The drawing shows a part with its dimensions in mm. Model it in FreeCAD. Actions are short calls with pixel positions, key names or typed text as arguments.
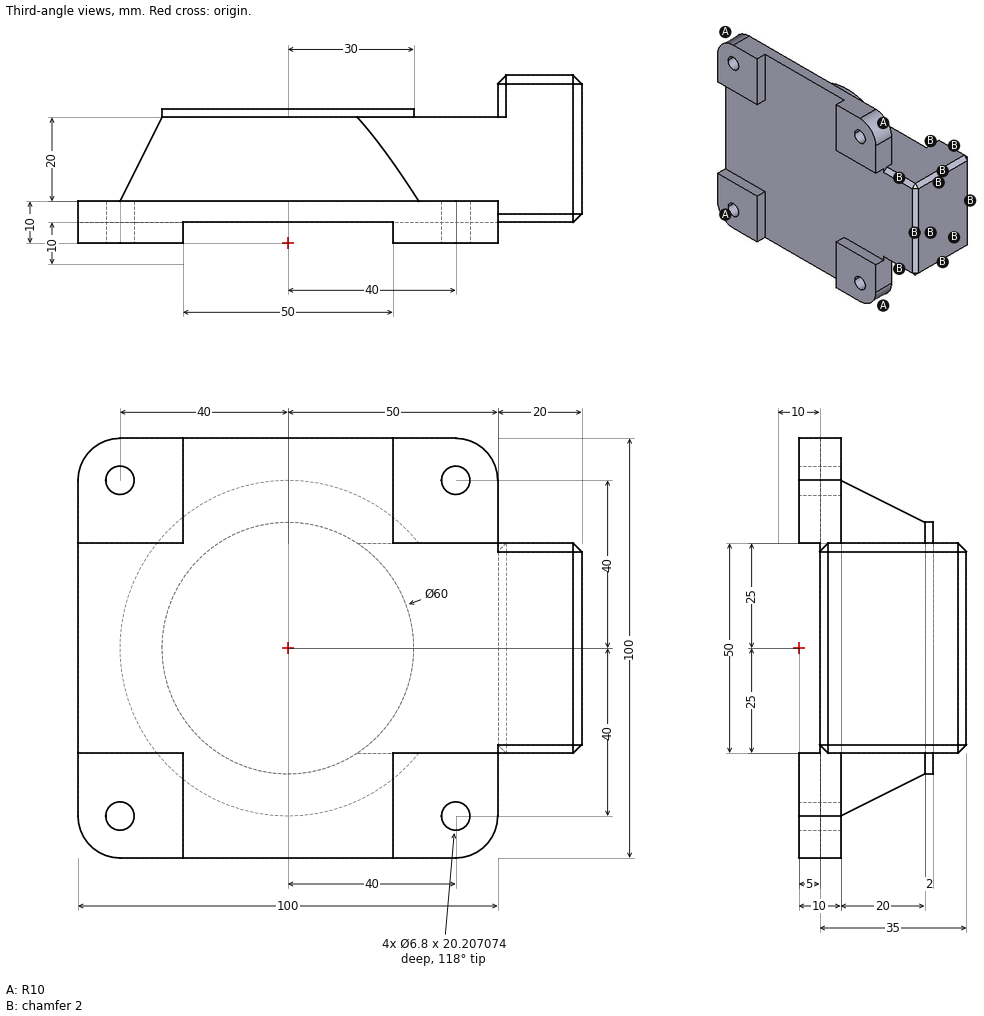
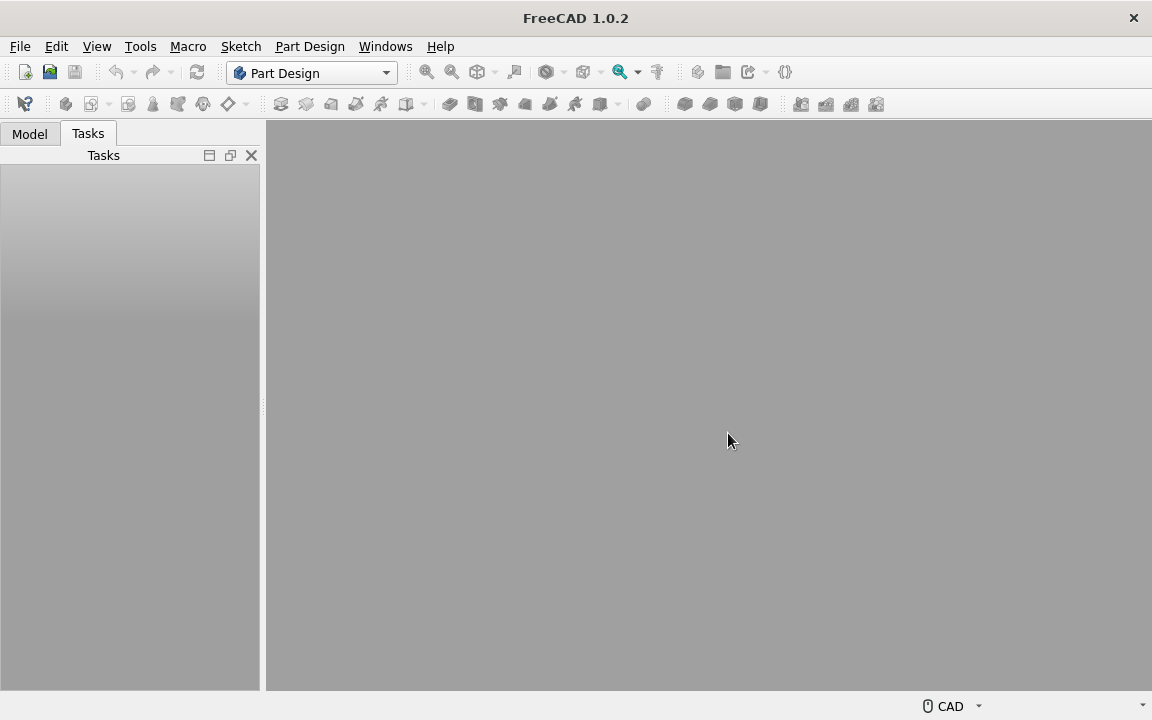
click(25, 72)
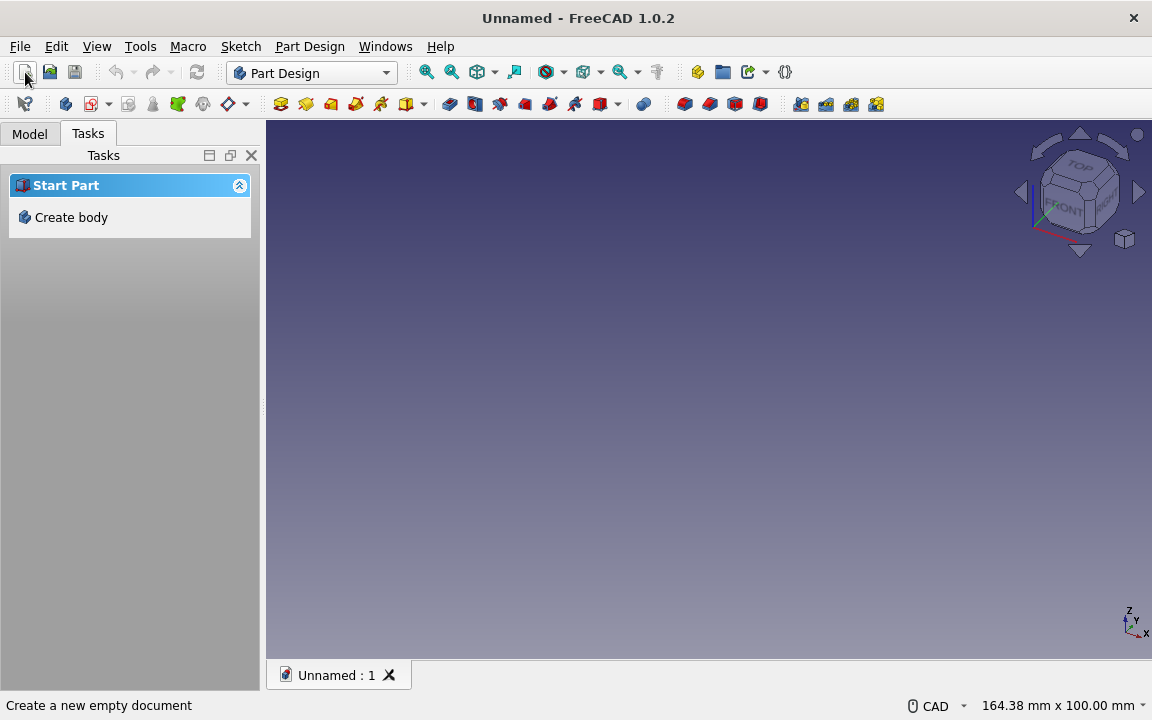
click(90, 104)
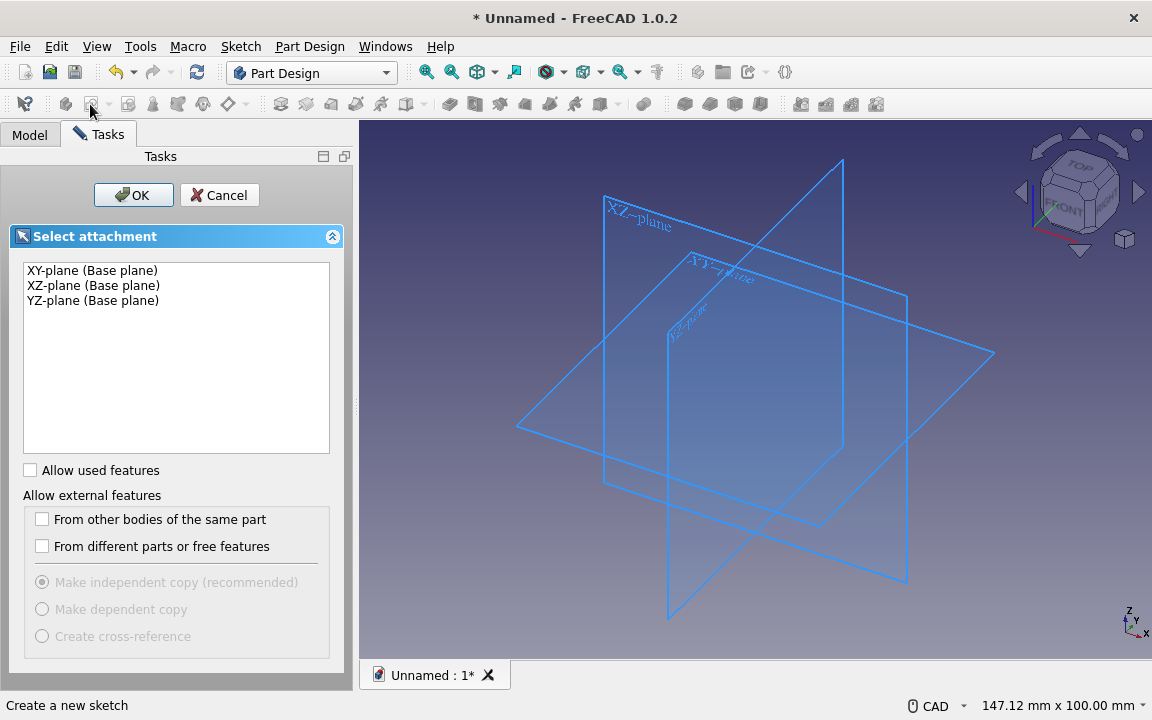
click(84, 286)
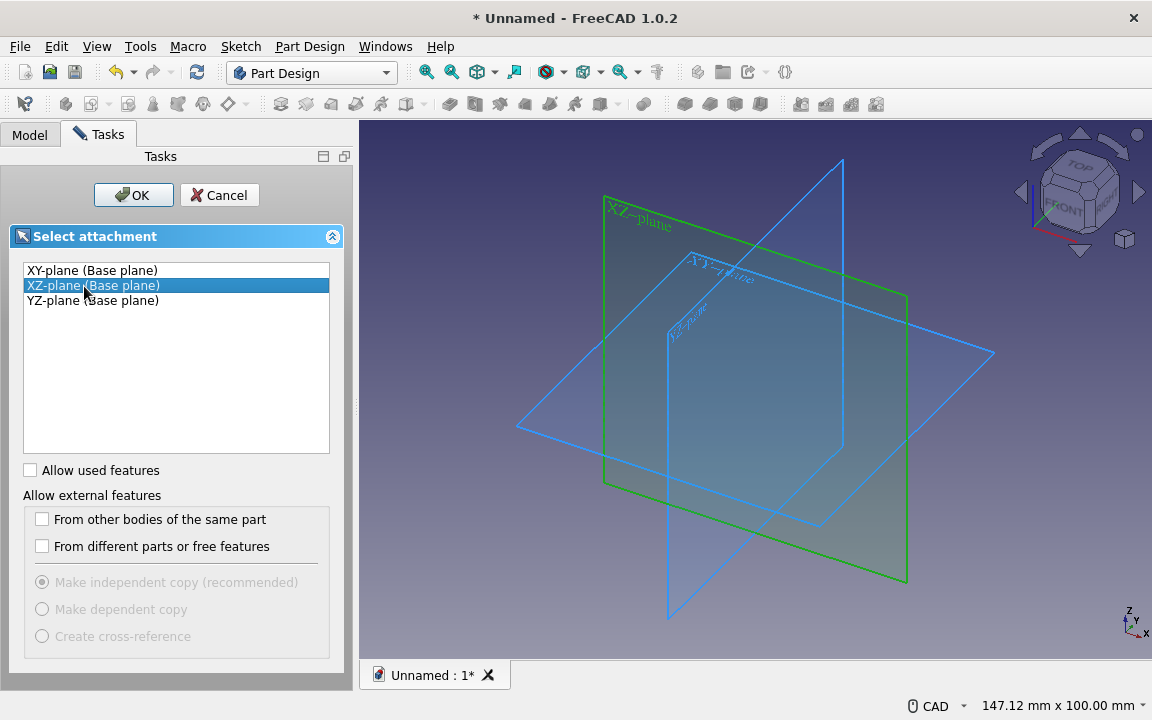
click(134, 195)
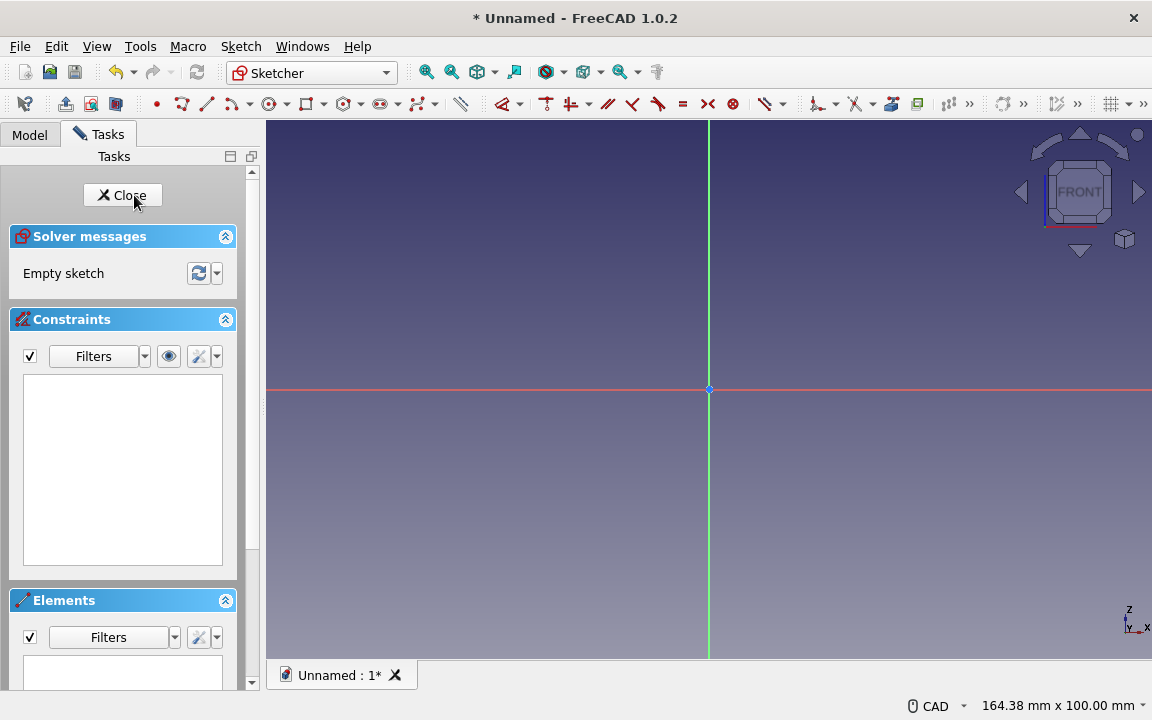
scroll(501, 390, down, 2)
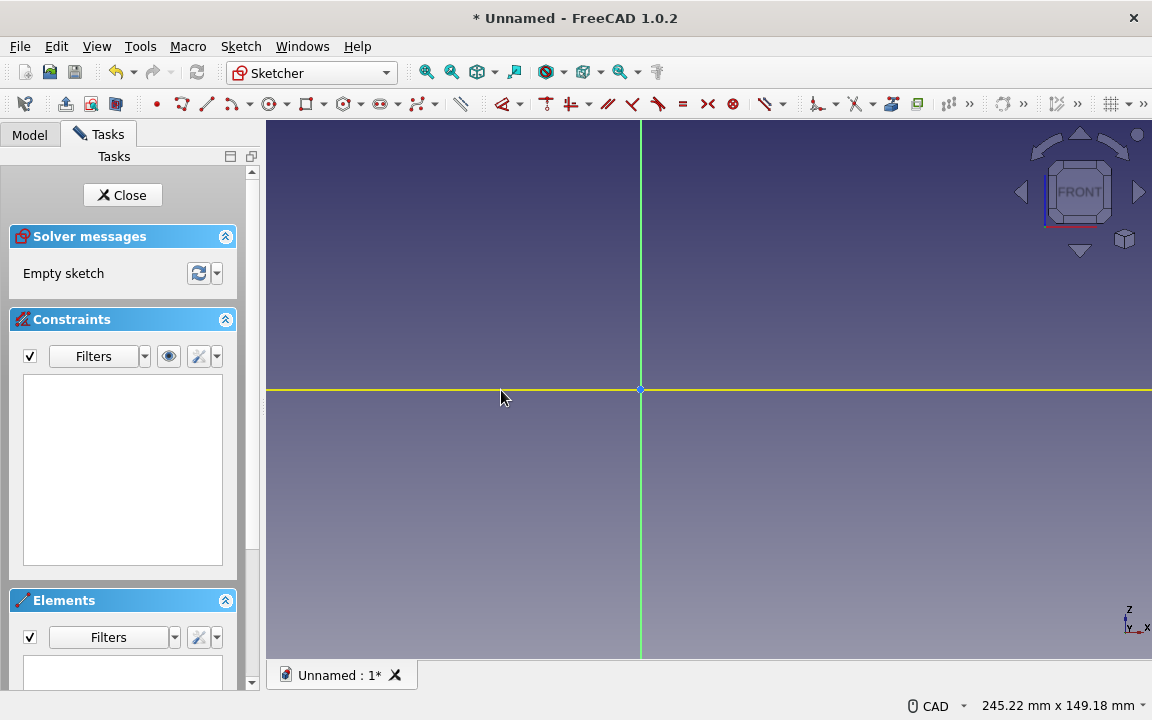
key(g)
key(v)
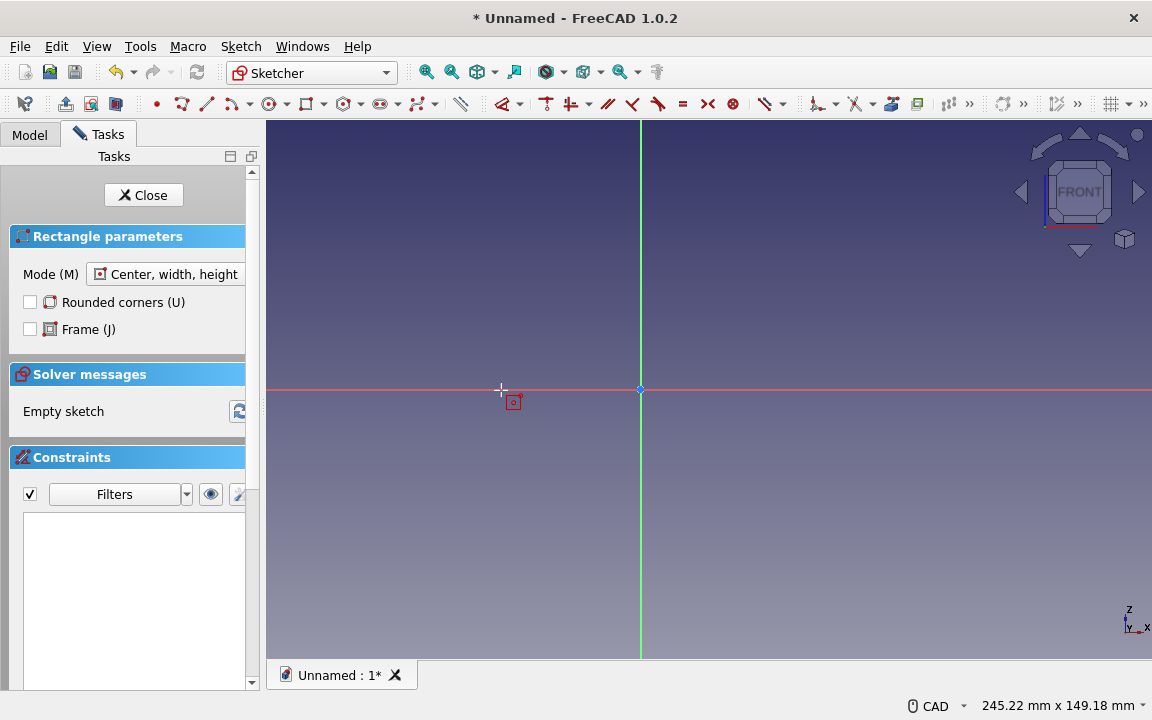
click(641, 390)
click(821, 209)
key(Escape)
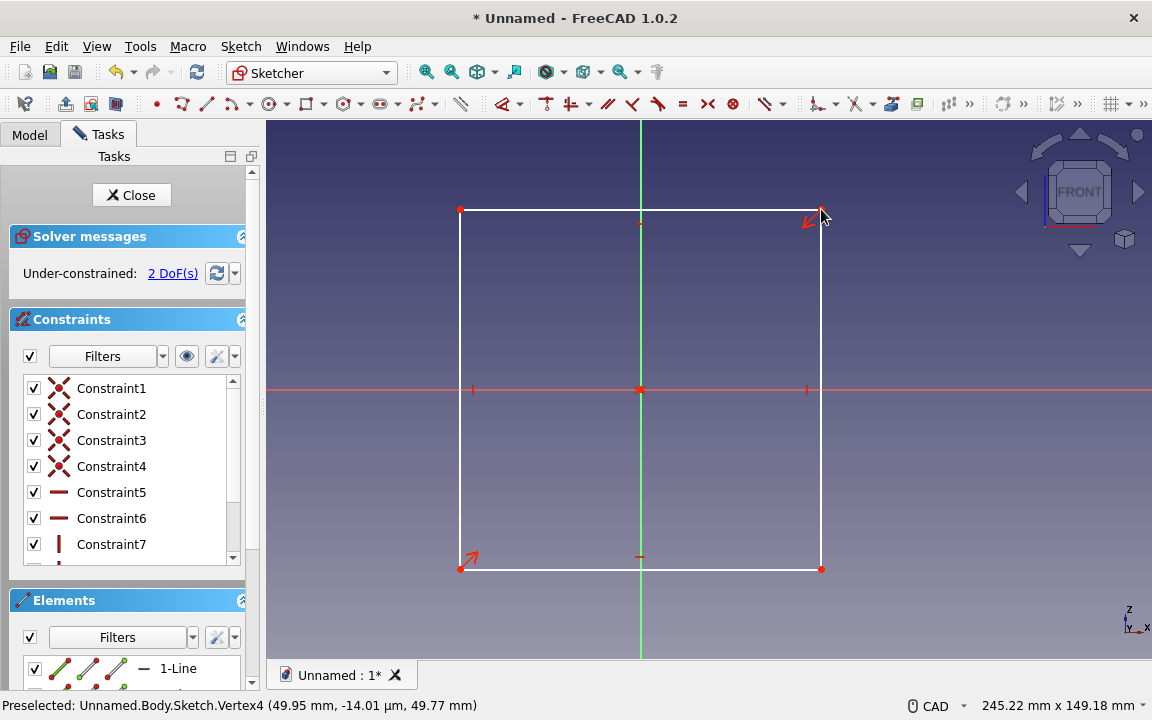
click(502, 104)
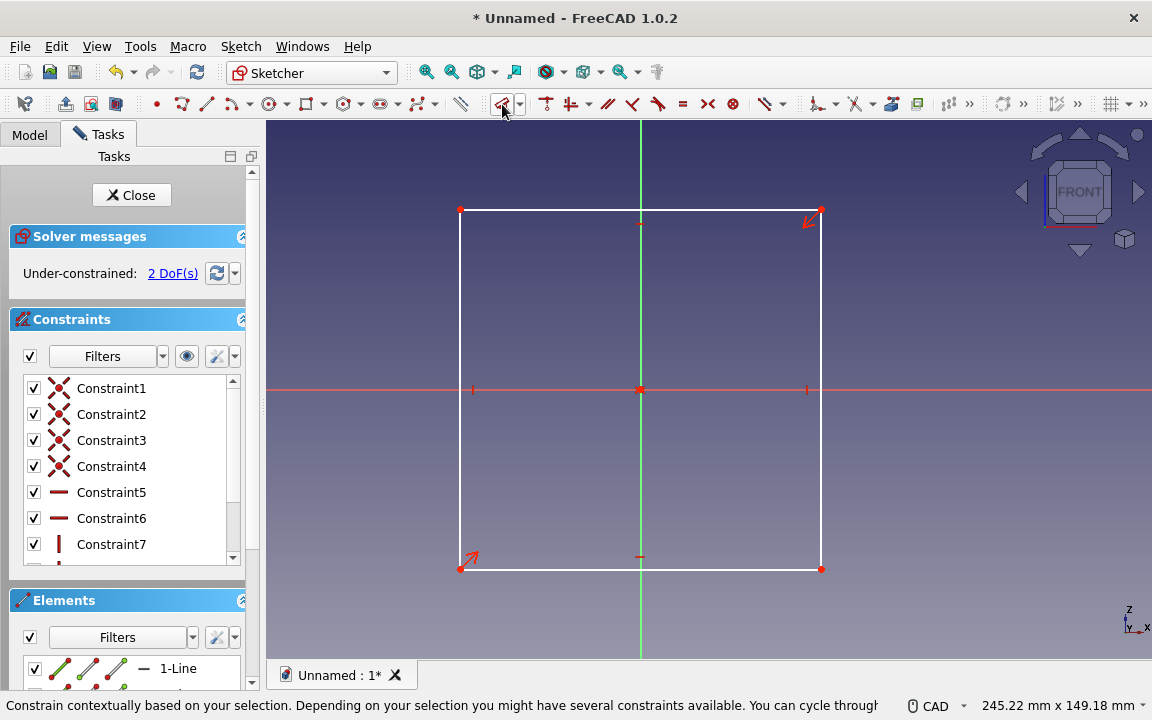
click(568, 570)
click(557, 604)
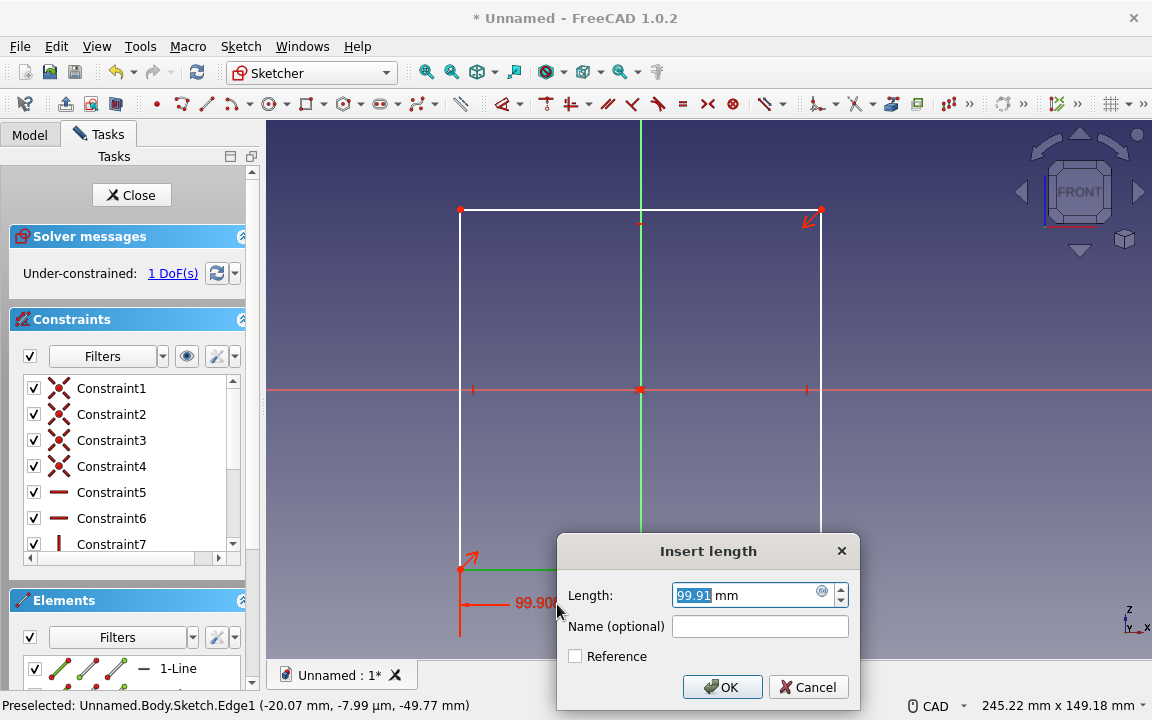
text(100)
key(Return)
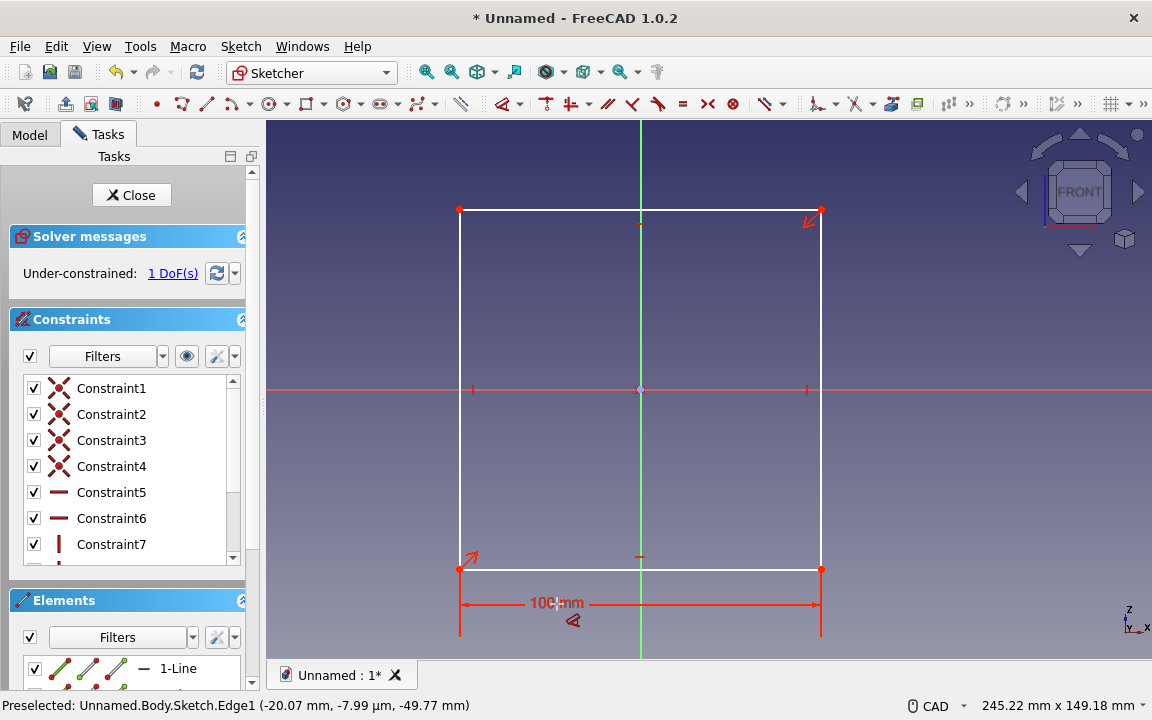
click(821, 462)
click(855, 307)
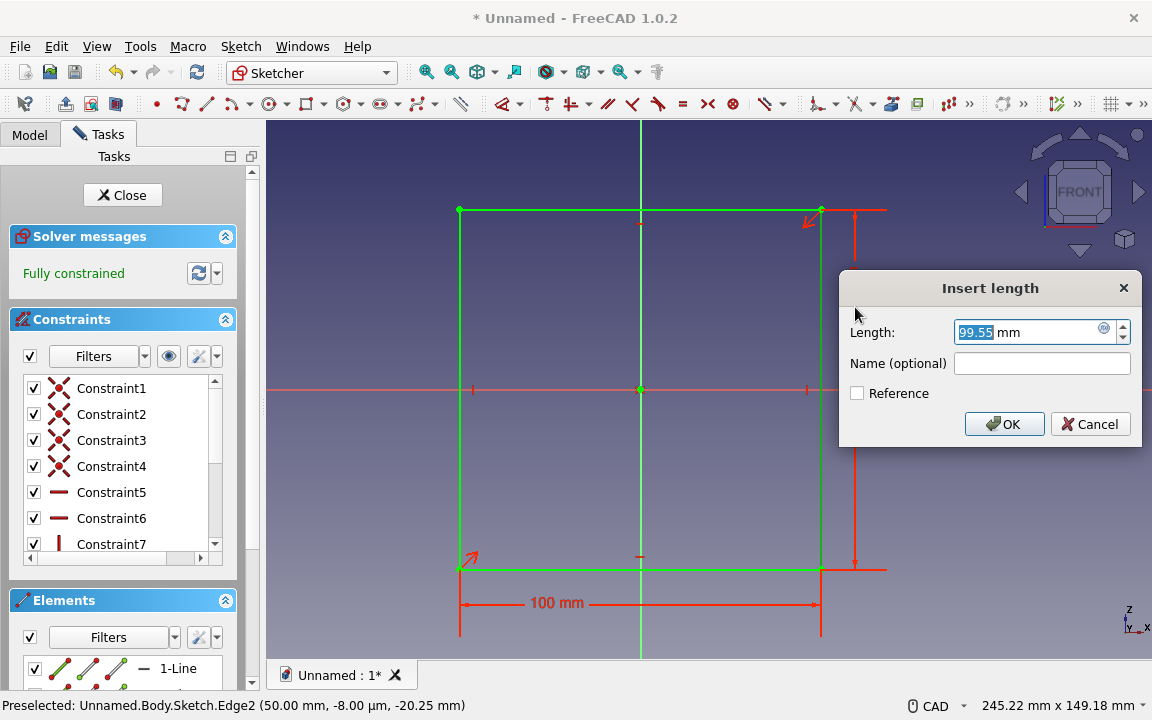
text(100)
key(Return)
key(Escape)